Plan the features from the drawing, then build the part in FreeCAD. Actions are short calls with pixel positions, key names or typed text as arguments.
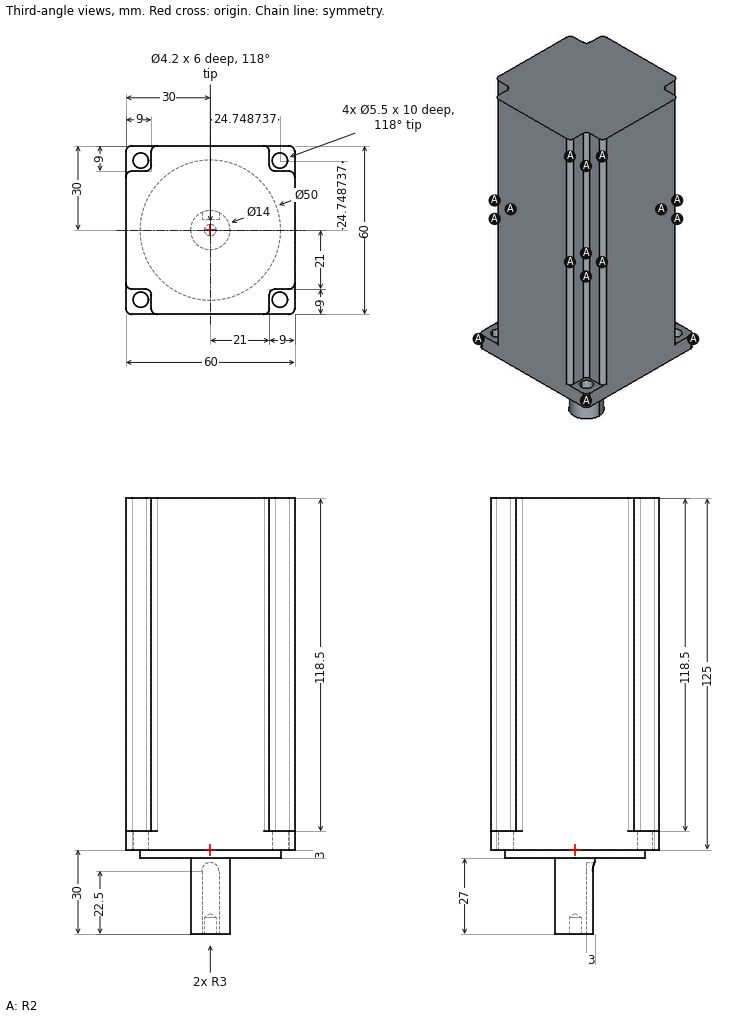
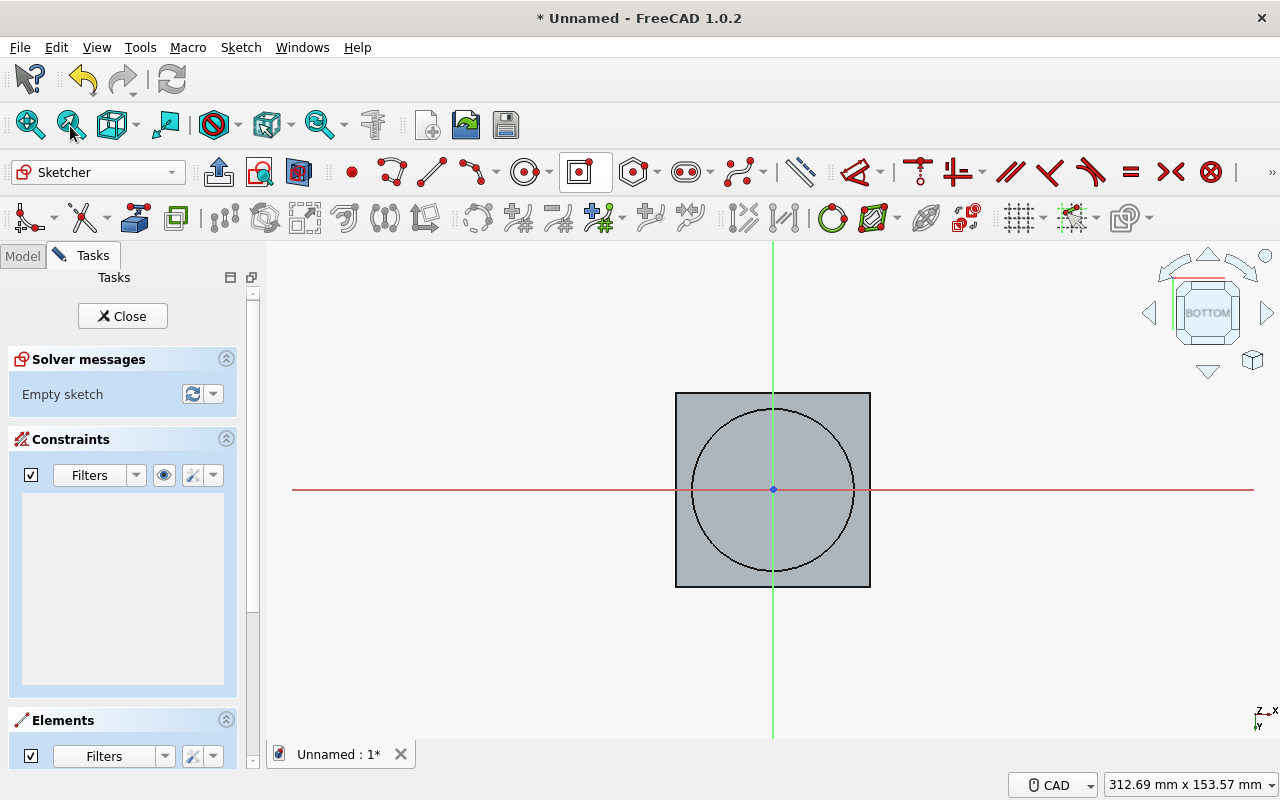
scroll(784, 490, up, 10)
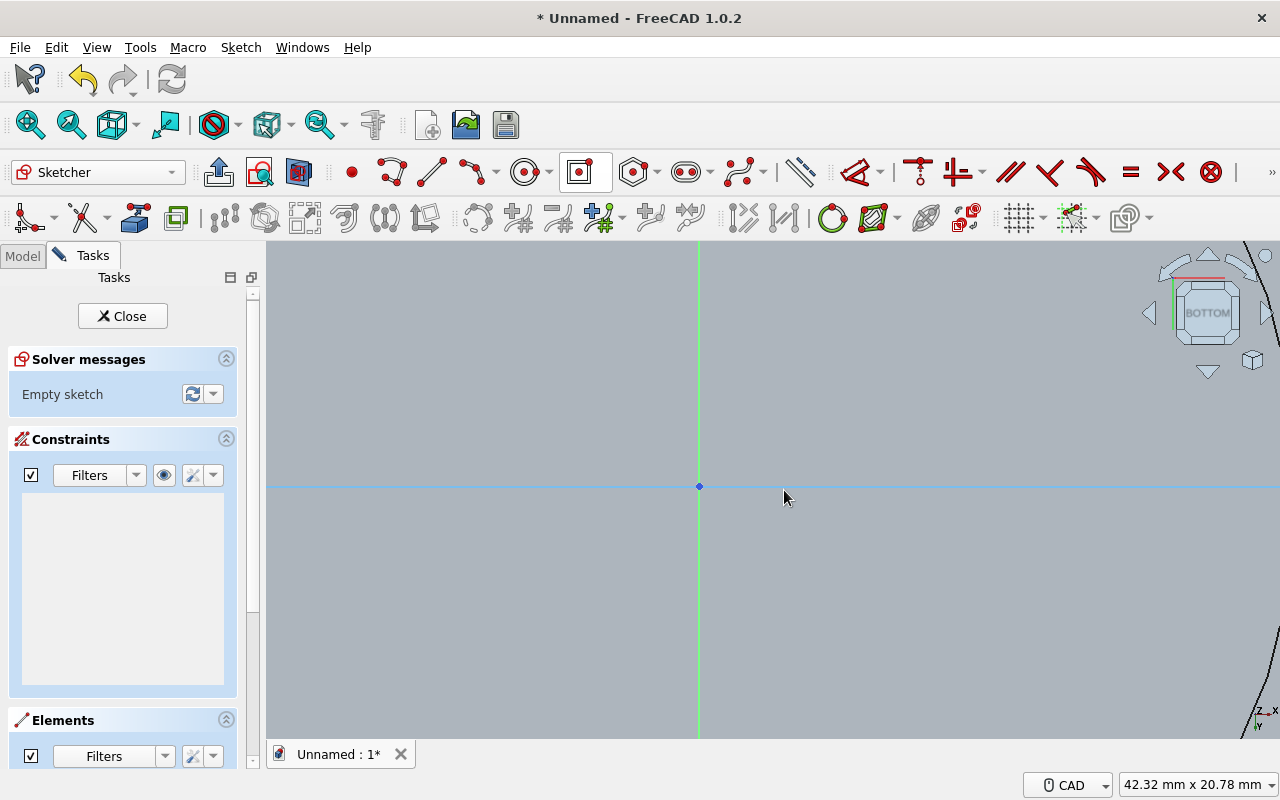
click(526, 172)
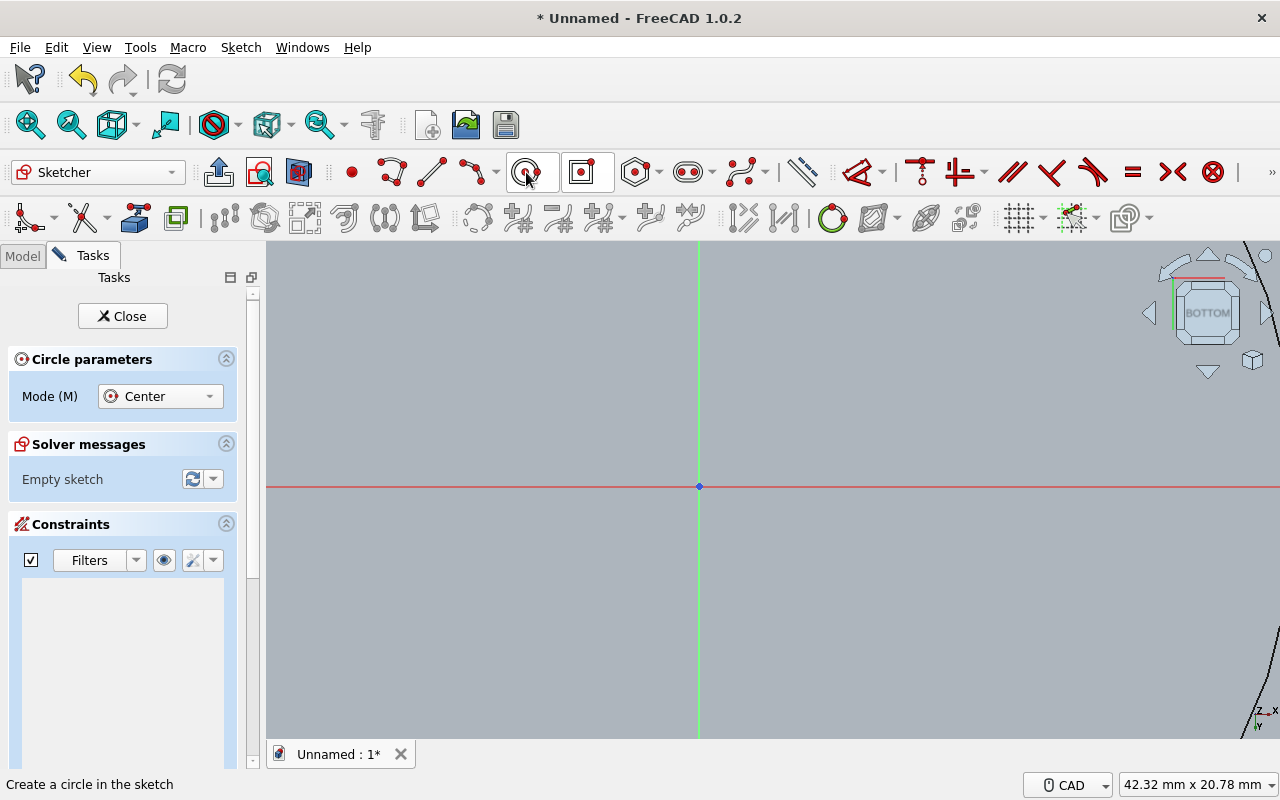
click(699, 487)
move(818, 368)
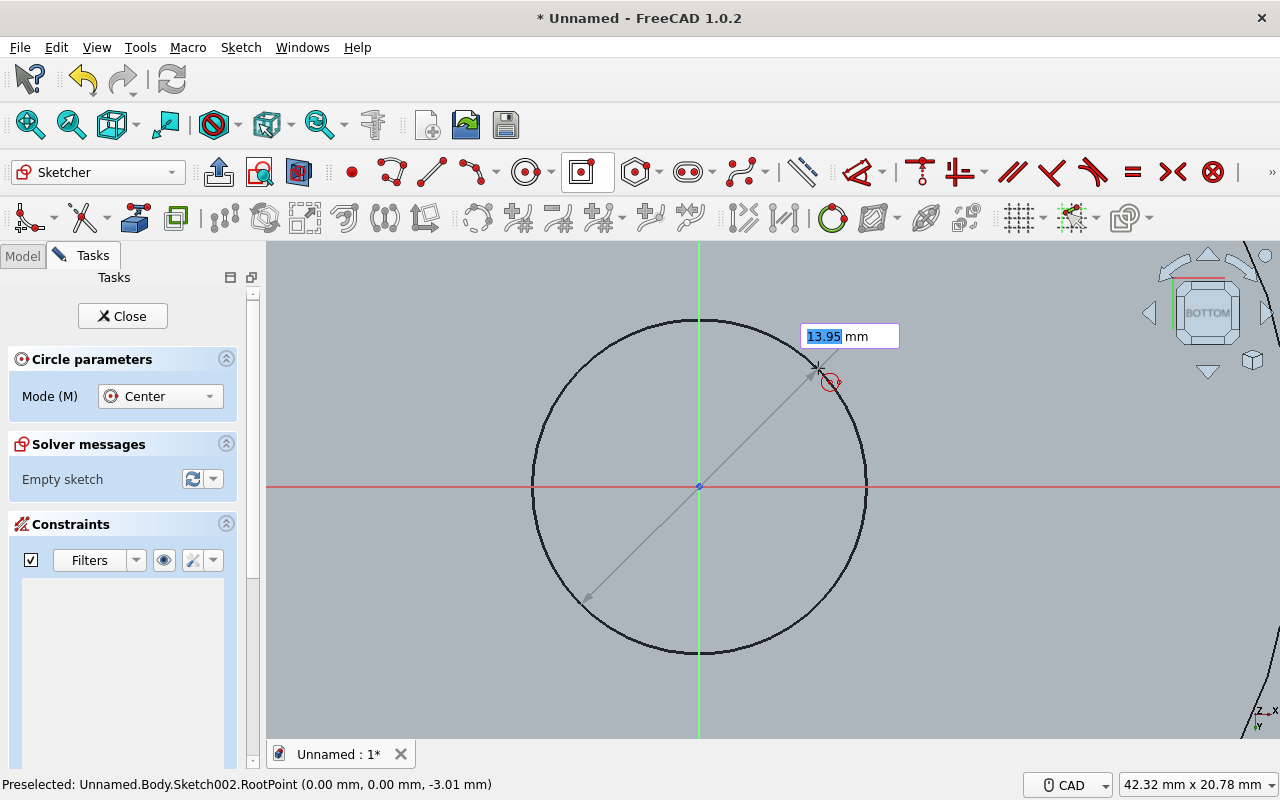
text(14)
key(Return)
key(Escape)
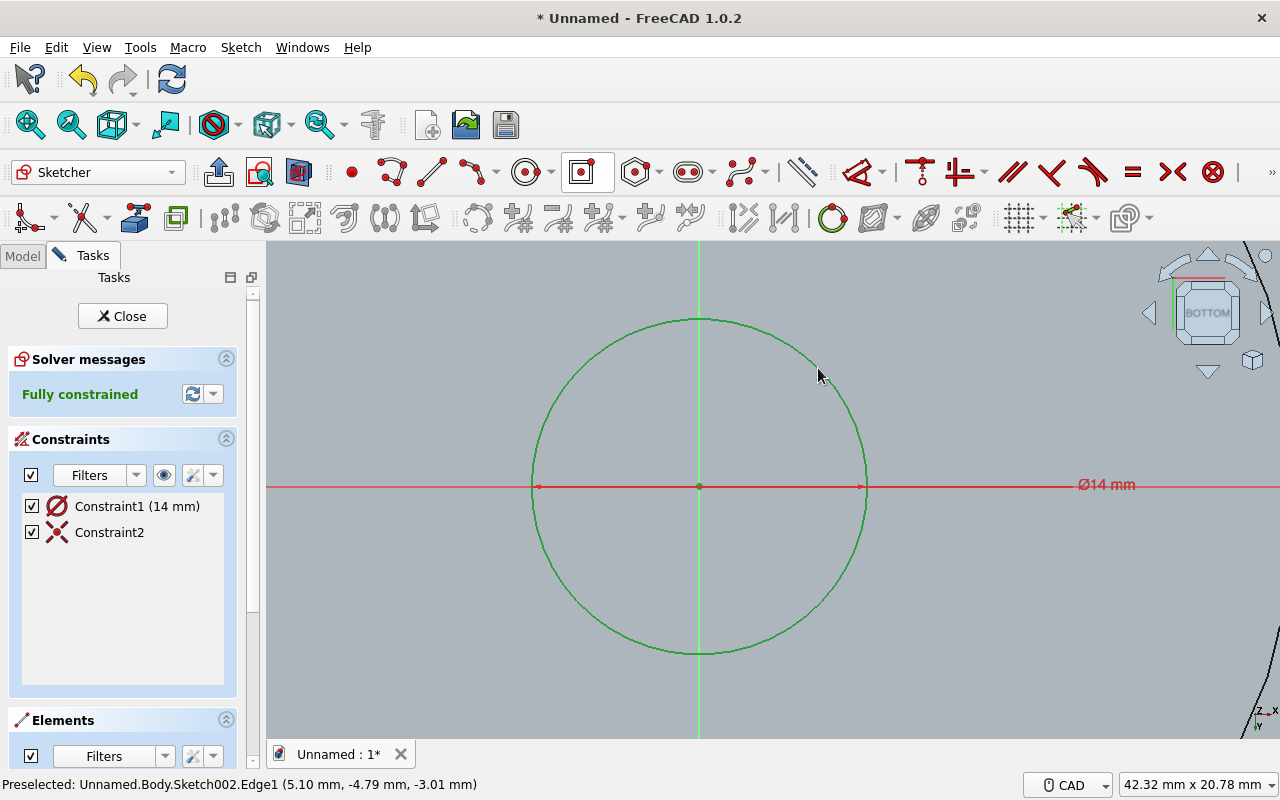
click(123, 316)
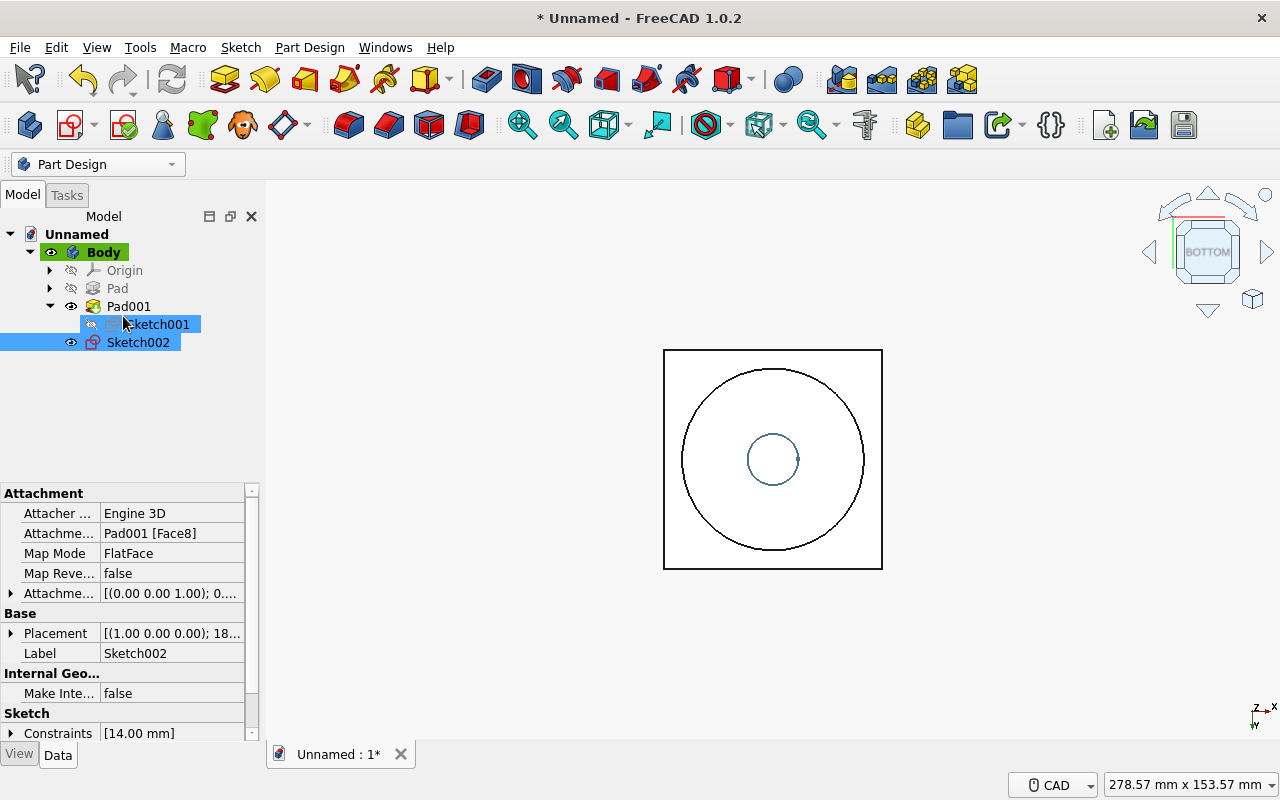
click(226, 80)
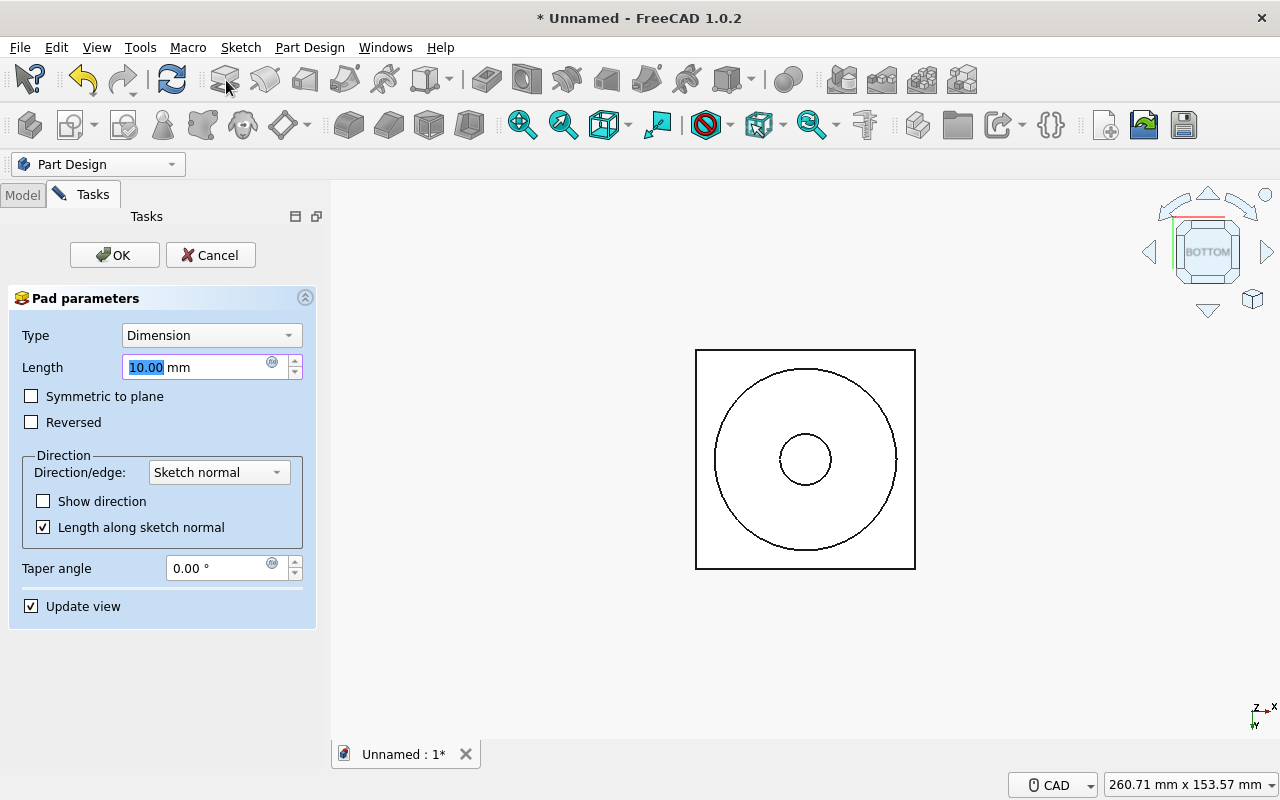
text(27)
key(Tab)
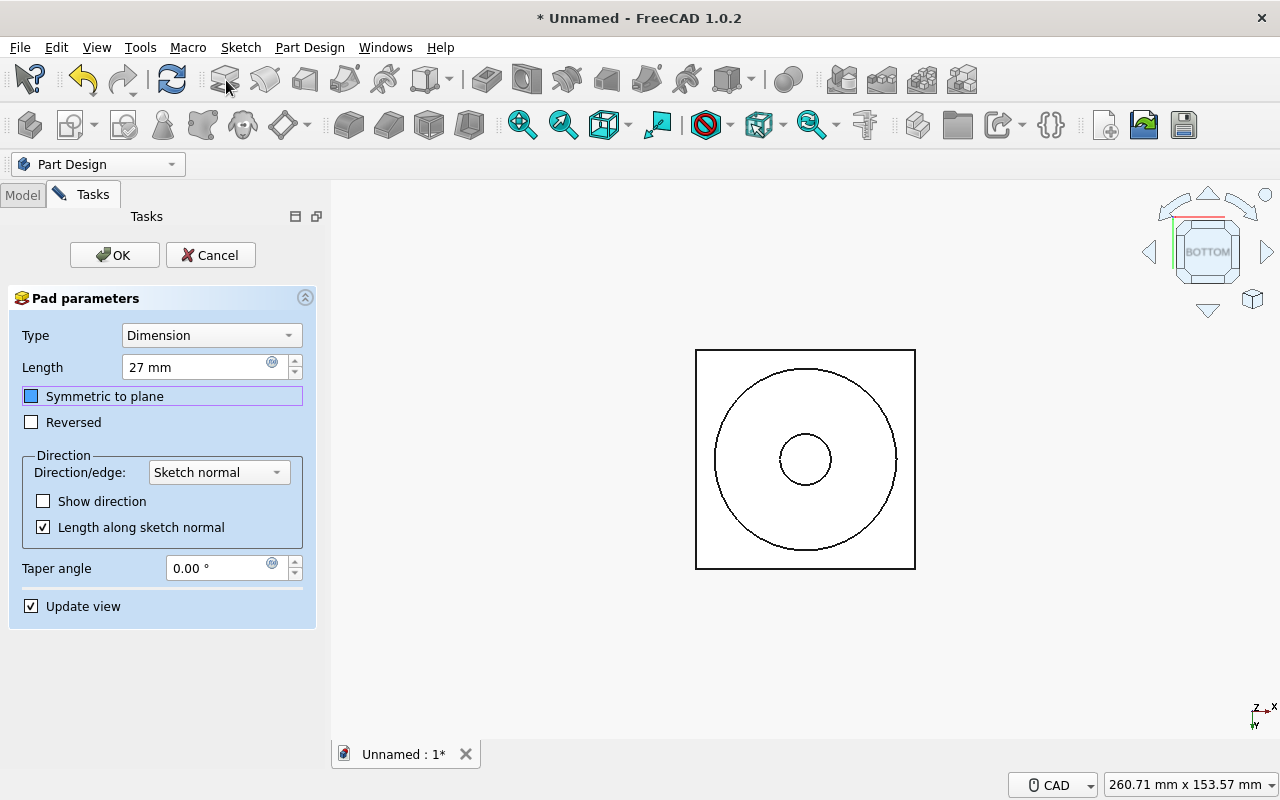
click(115, 255)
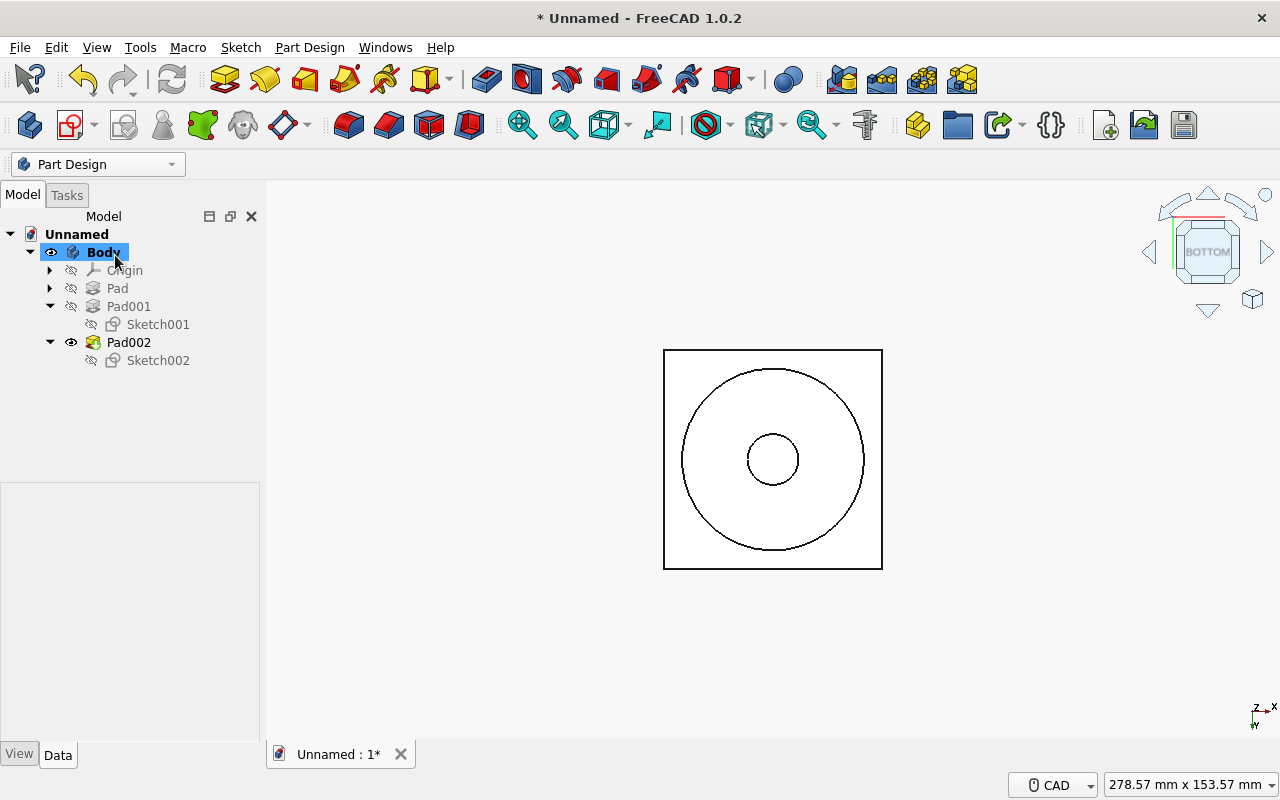
click(524, 126)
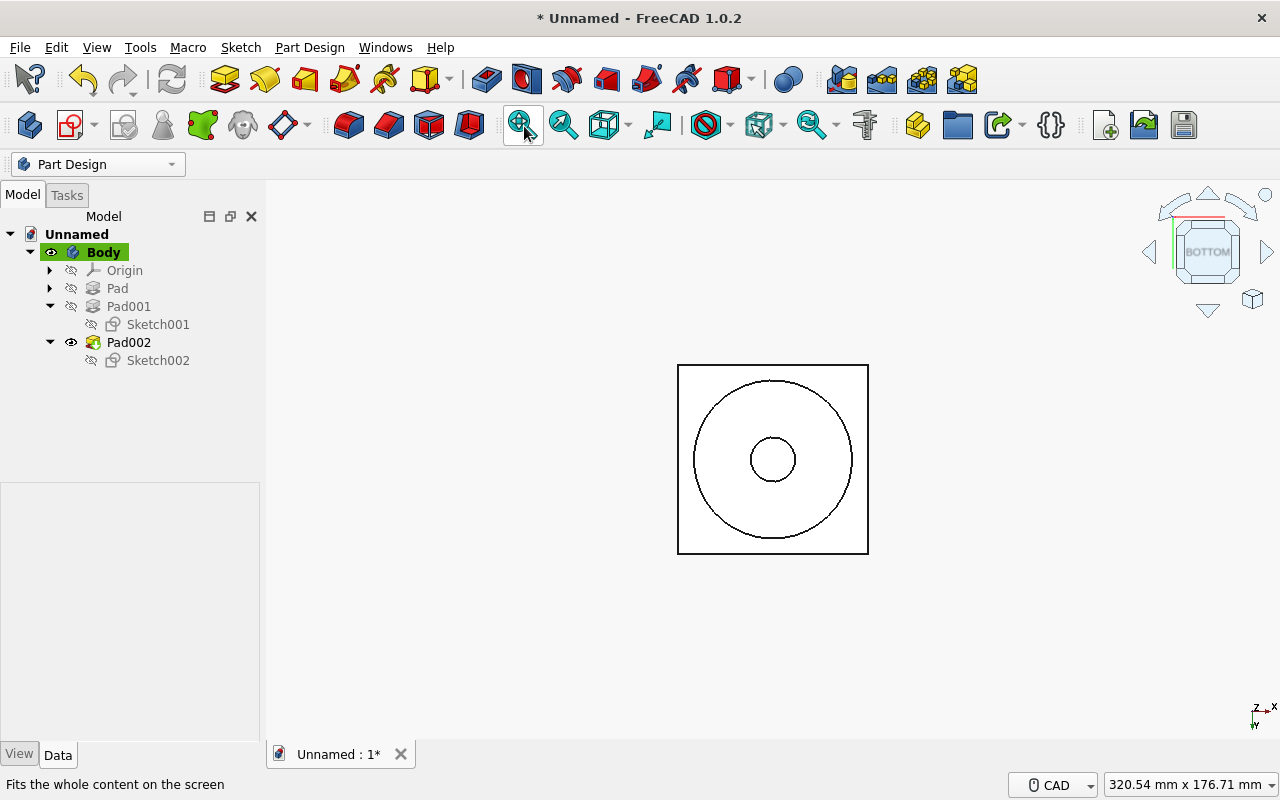
click(50, 270)